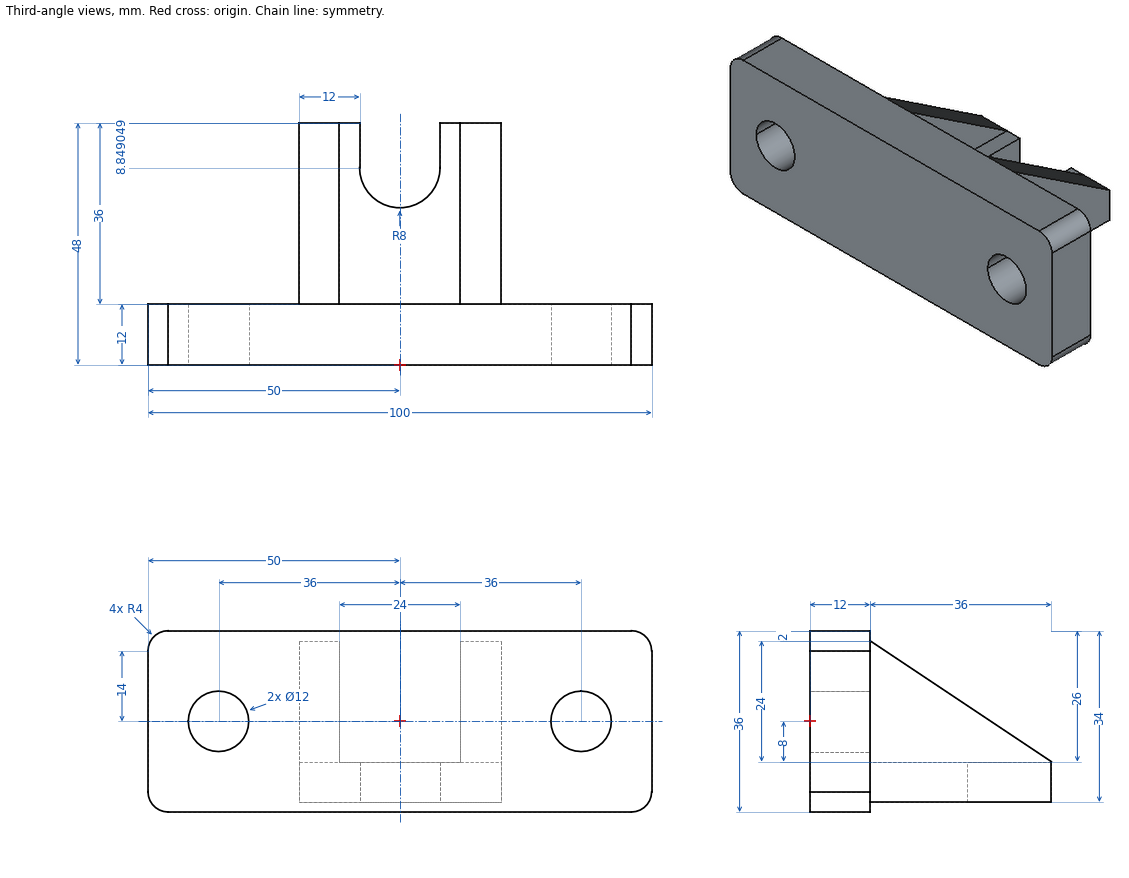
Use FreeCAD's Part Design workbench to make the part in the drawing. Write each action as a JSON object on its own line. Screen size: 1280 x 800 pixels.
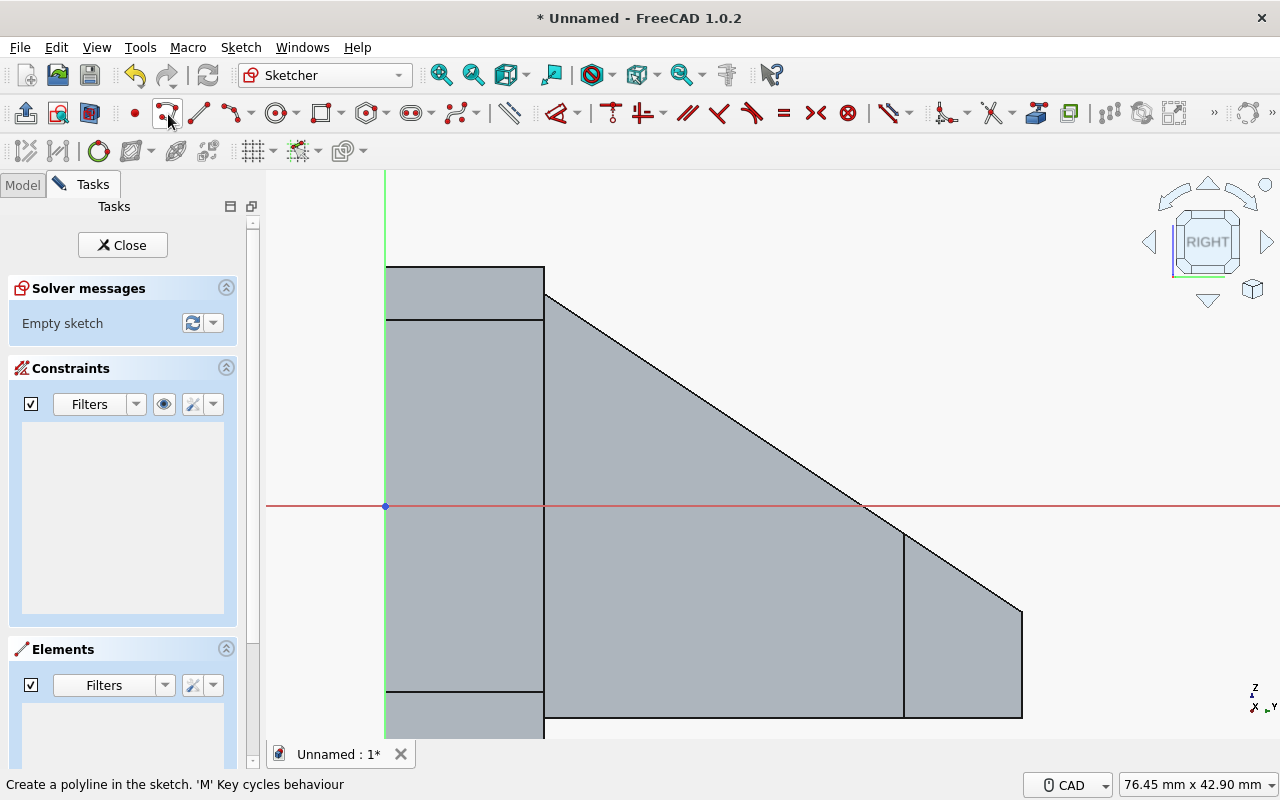
{"action": "left_click", "coordinate": [544, 612]}
{"action": "left_click", "coordinate": [1022, 612]}
{"action": "left_click", "coordinate": [544, 294]}
{"action": "left_click", "coordinate": [544, 613]}
{"action": "key", "text": "Escape"}
{"action": "key", "text": "Escape"}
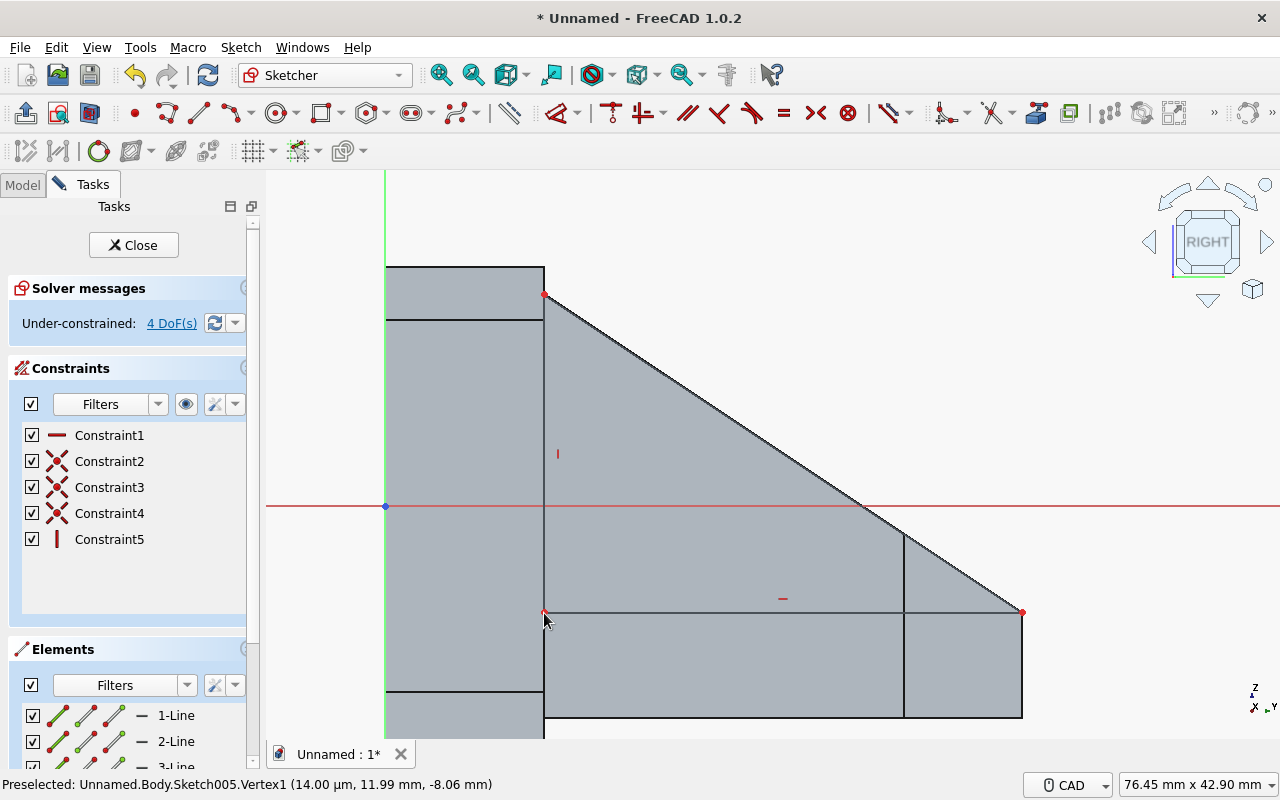
{"action": "left_click", "coordinate": [556, 114]}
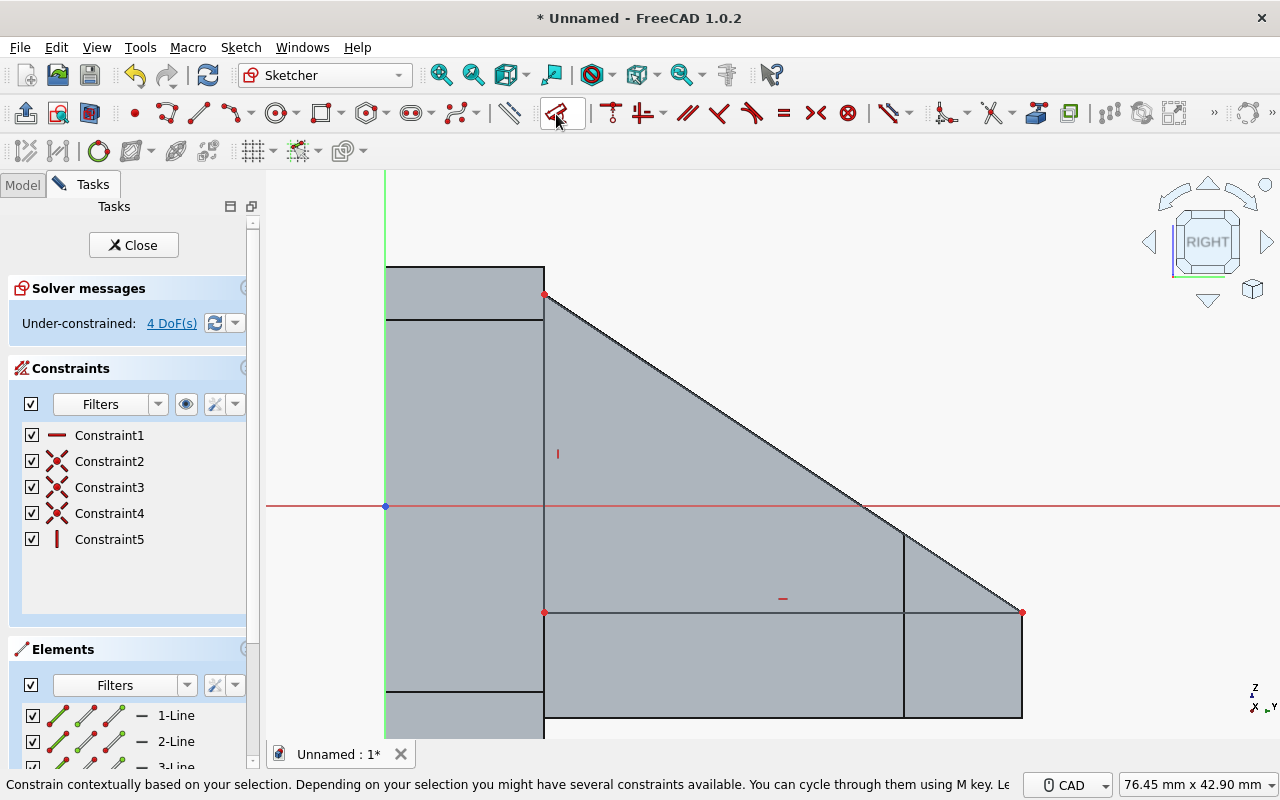
{"action": "left_click", "coordinate": [687, 613]}
{"action": "left_click", "coordinate": [783, 647]}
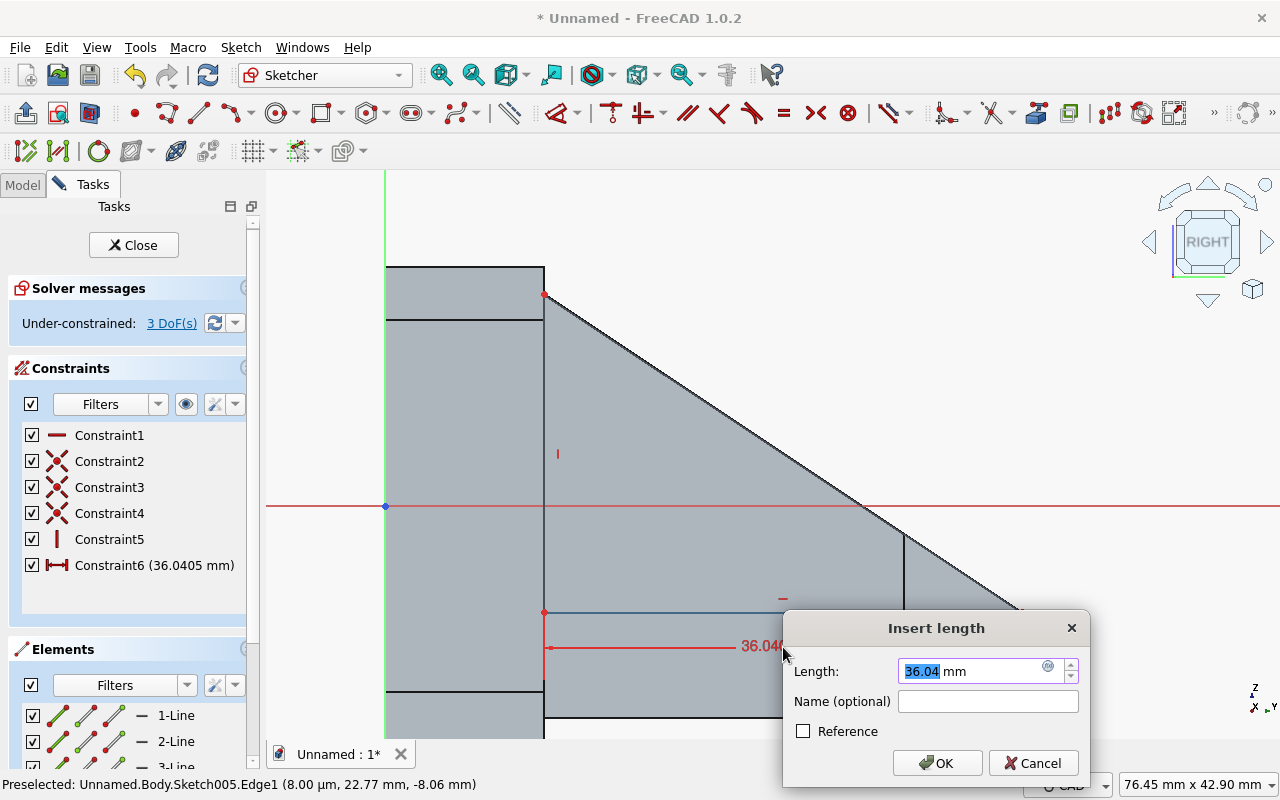
{"action": "type", "text": "36"}
{"action": "key", "text": "Return"}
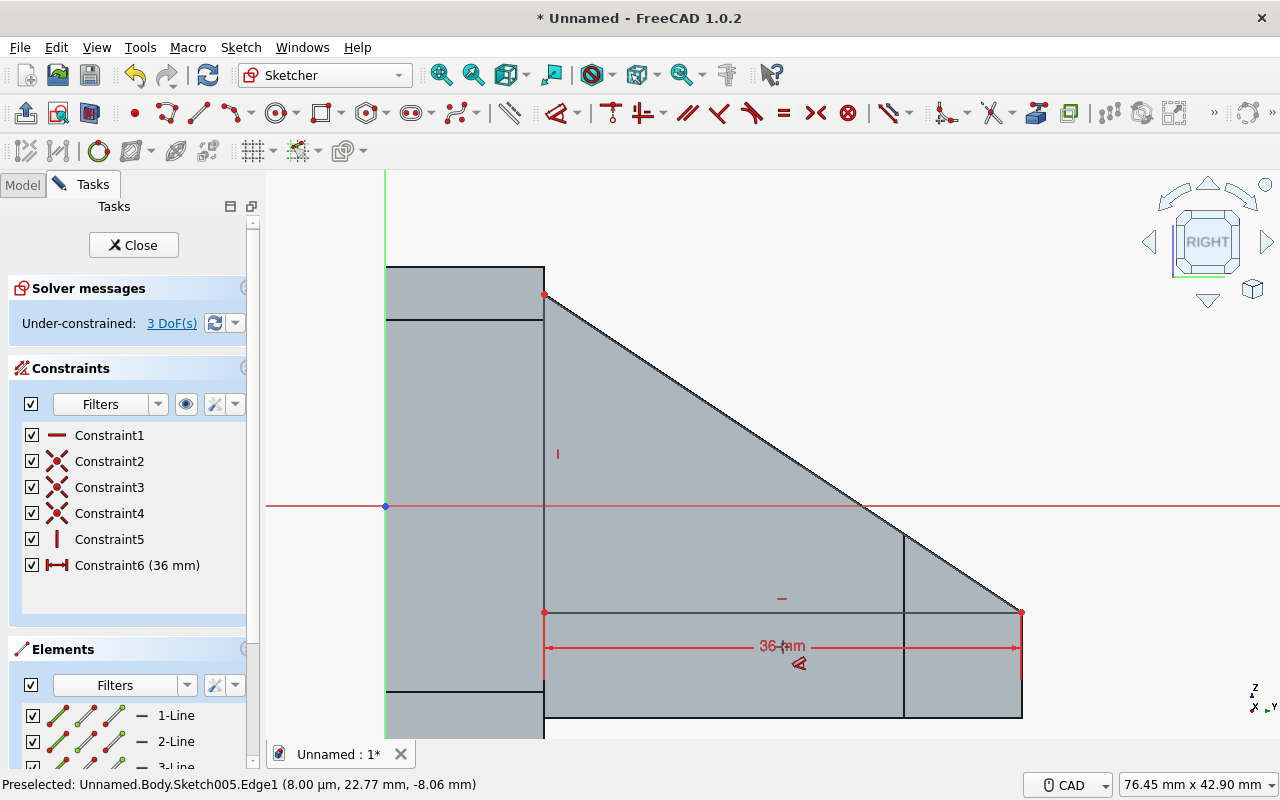
{"action": "left_click", "coordinate": [544, 390]}
{"action": "left_click", "coordinate": [510, 454]}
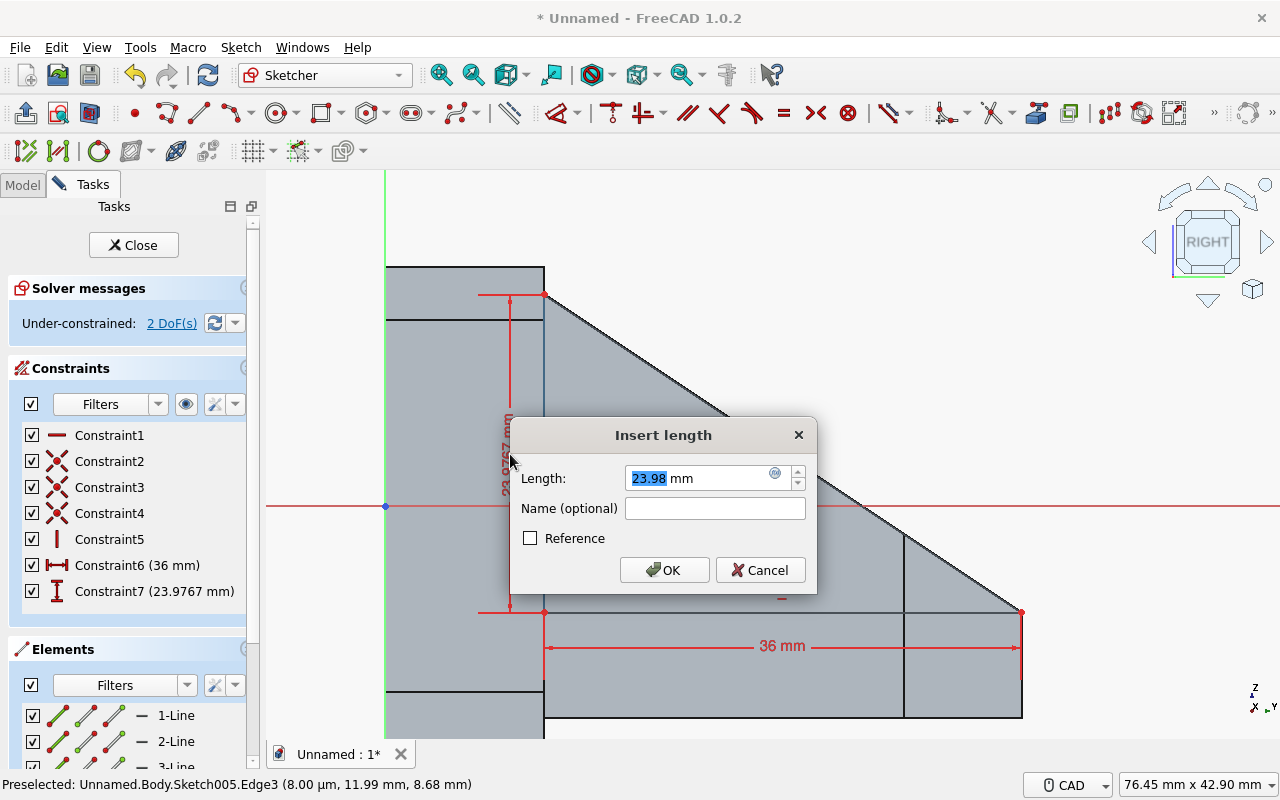
{"action": "type", "text": "24"}
{"action": "key", "text": "Return"}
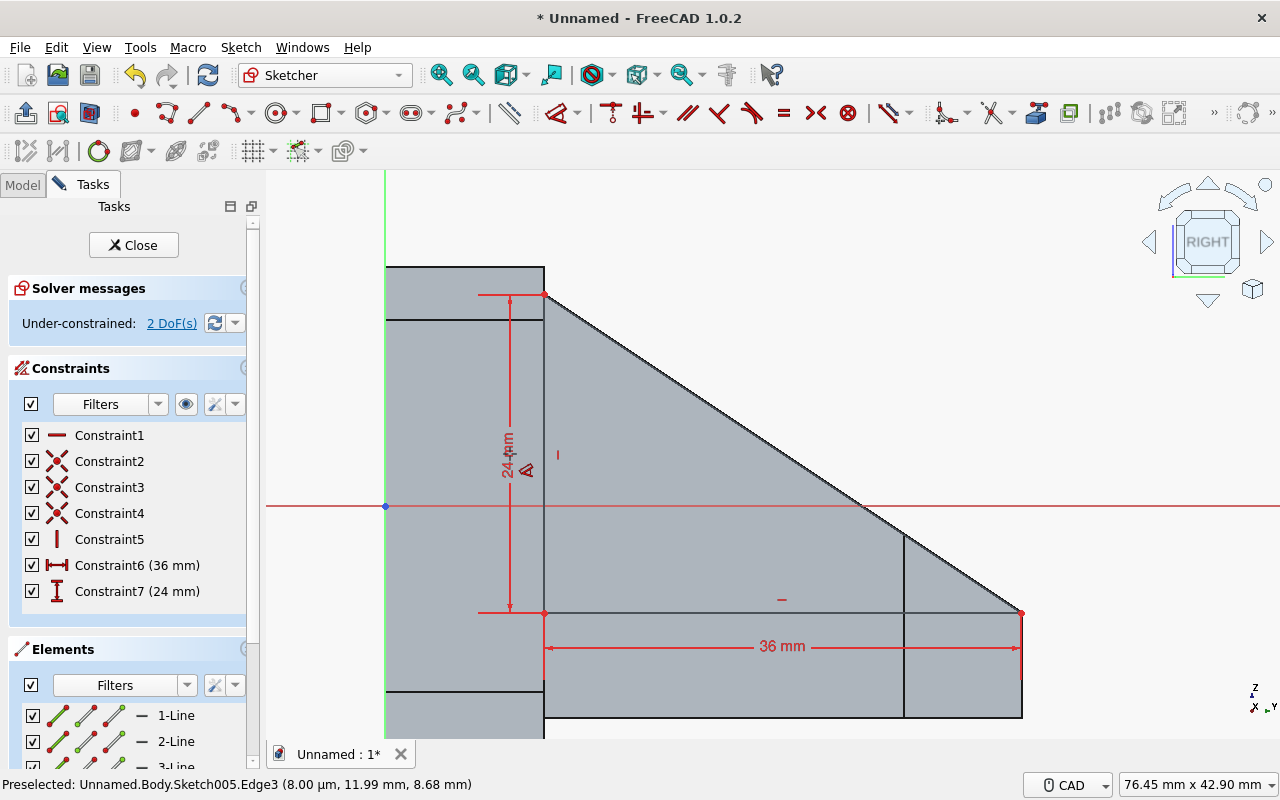
{"action": "left_click", "coordinate": [544, 613]}
{"action": "left_click", "coordinate": [351, 560]}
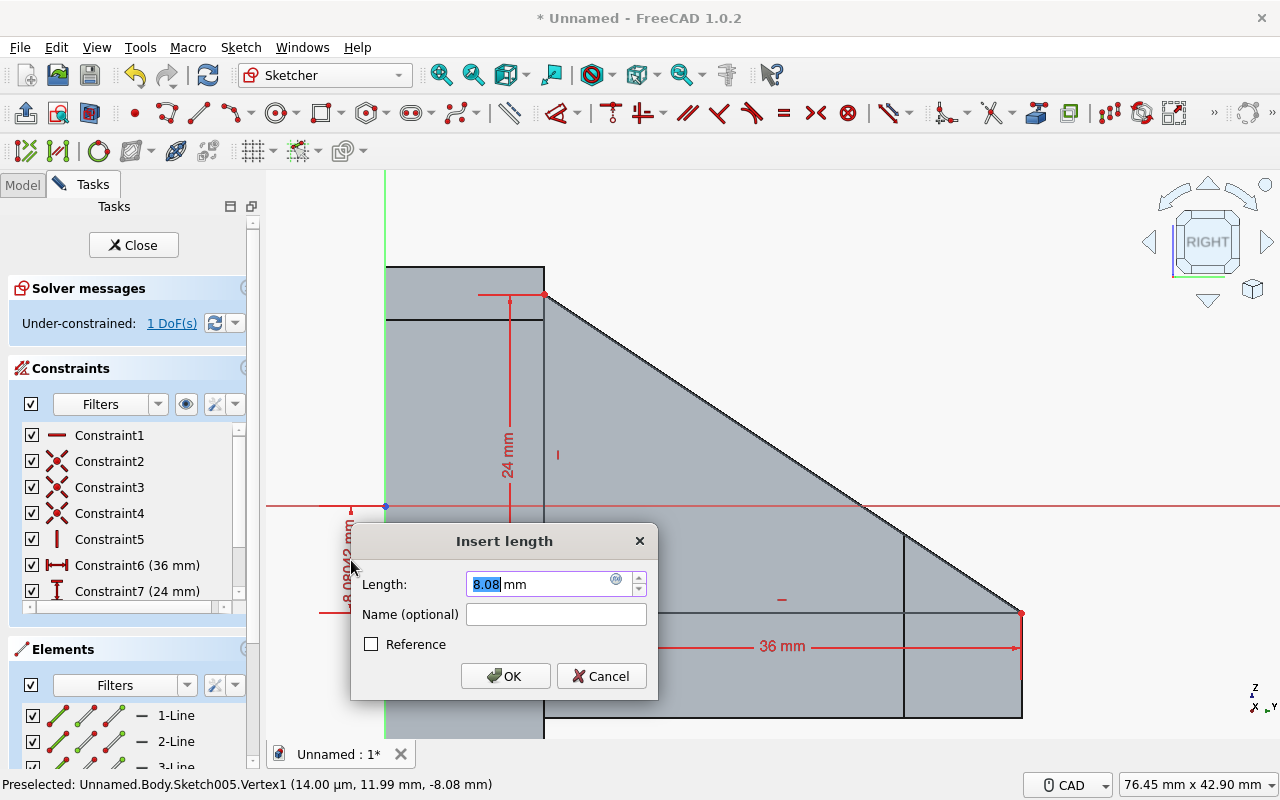
{"action": "type", "text": "8"}
{"action": "key", "text": "Return"}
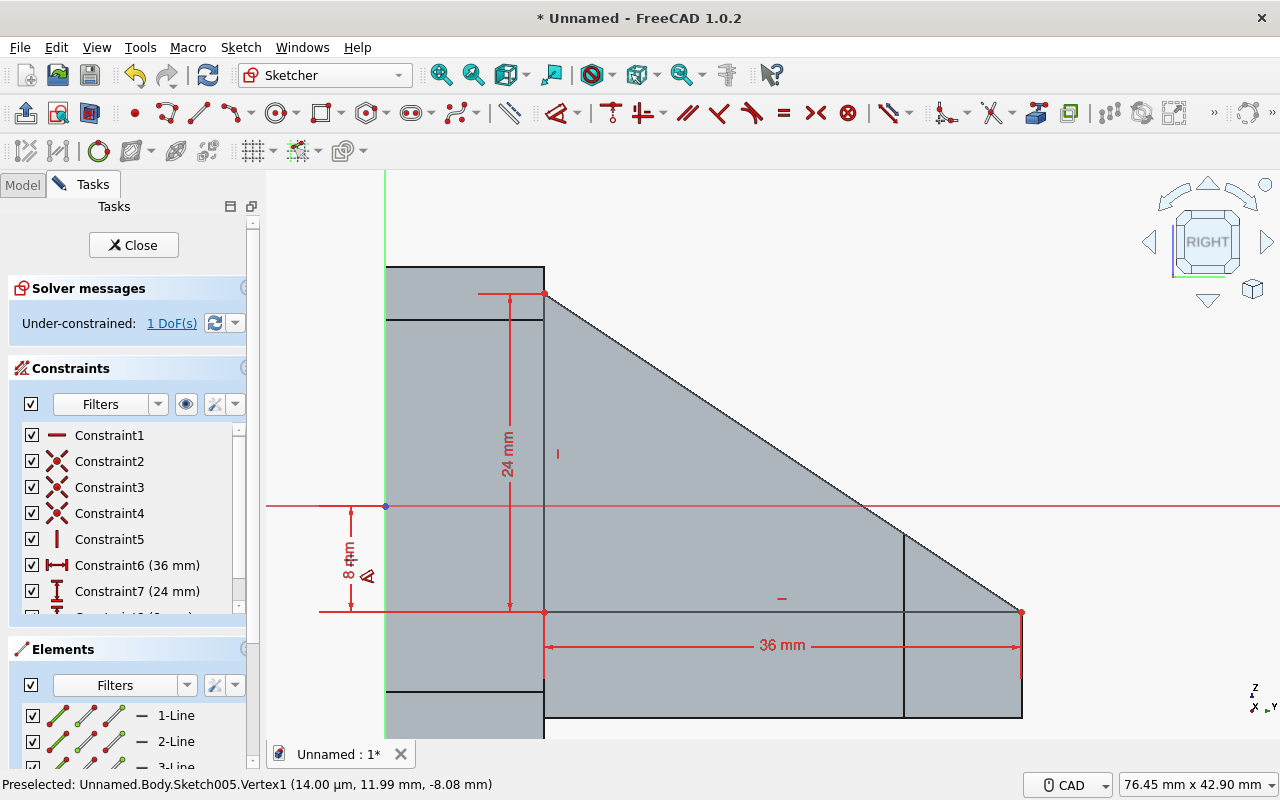
{"action": "left_click", "coordinate": [544, 612]}
{"action": "left_click", "coordinate": [465, 646]}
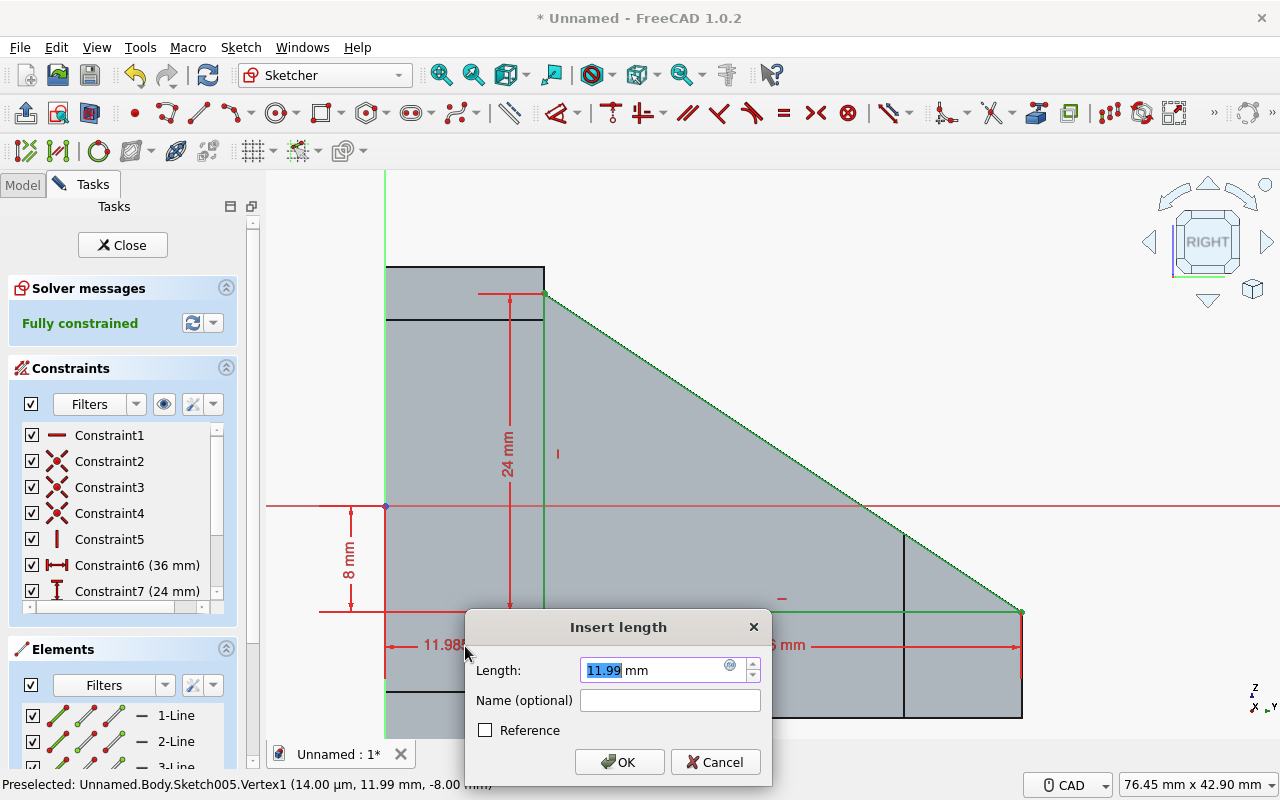
{"action": "type", "text": "12"}
{"action": "key", "text": "Return"}
{"action": "key", "text": "Escape"}